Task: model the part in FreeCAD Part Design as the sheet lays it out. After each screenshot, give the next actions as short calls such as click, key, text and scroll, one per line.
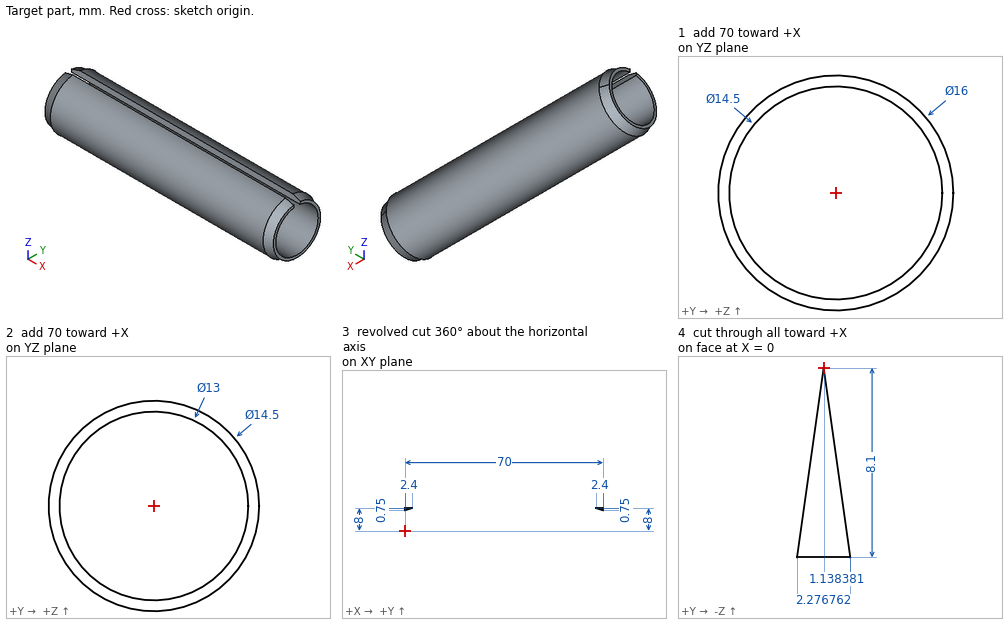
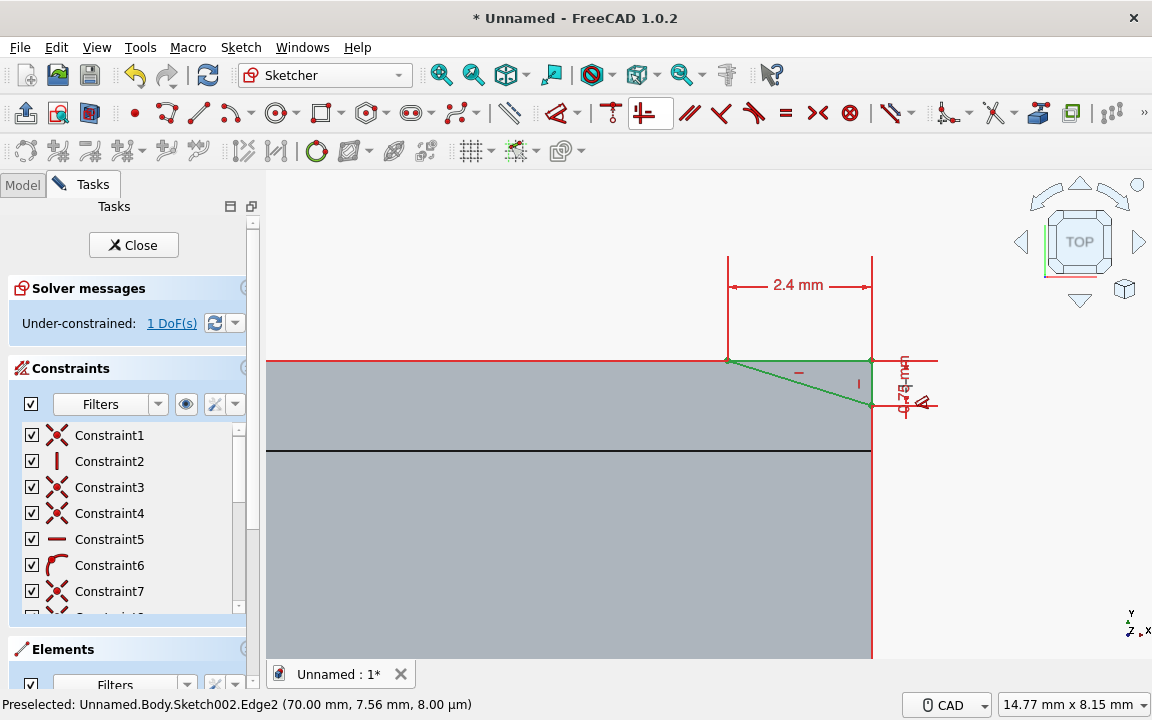
scroll(873, 391, down, 11)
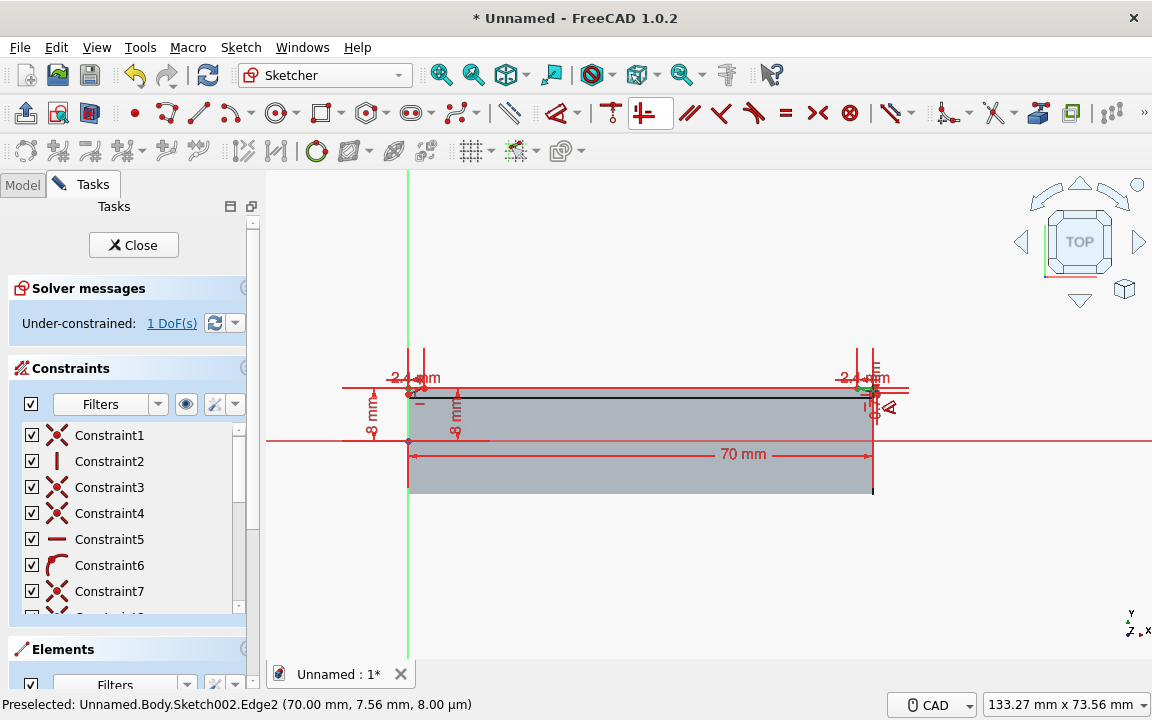
scroll(408, 390, up, 11)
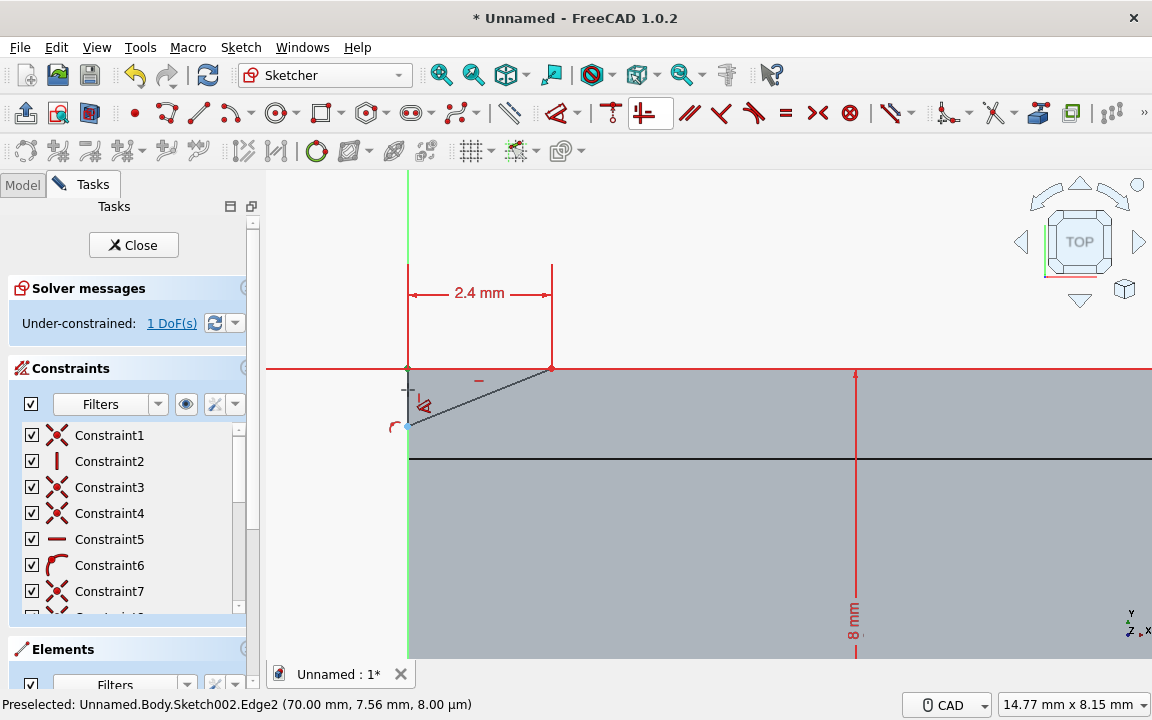
click(408, 386)
click(374, 398)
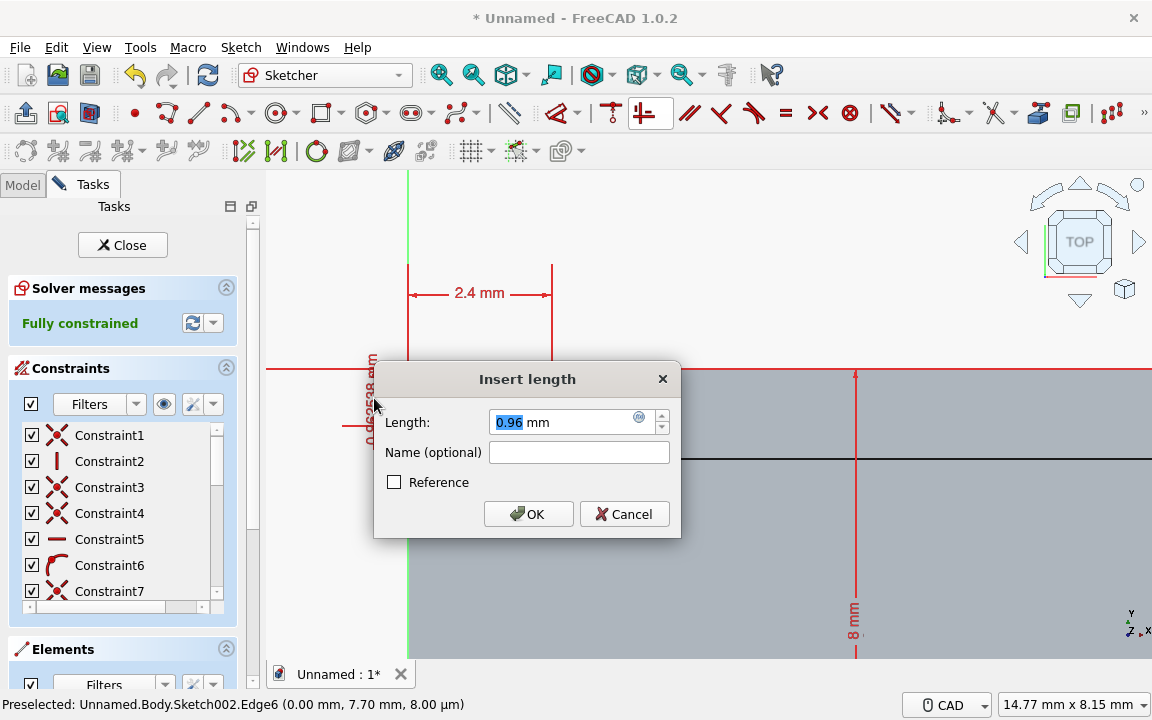
text(0.75)
key(Return)
key(Escape)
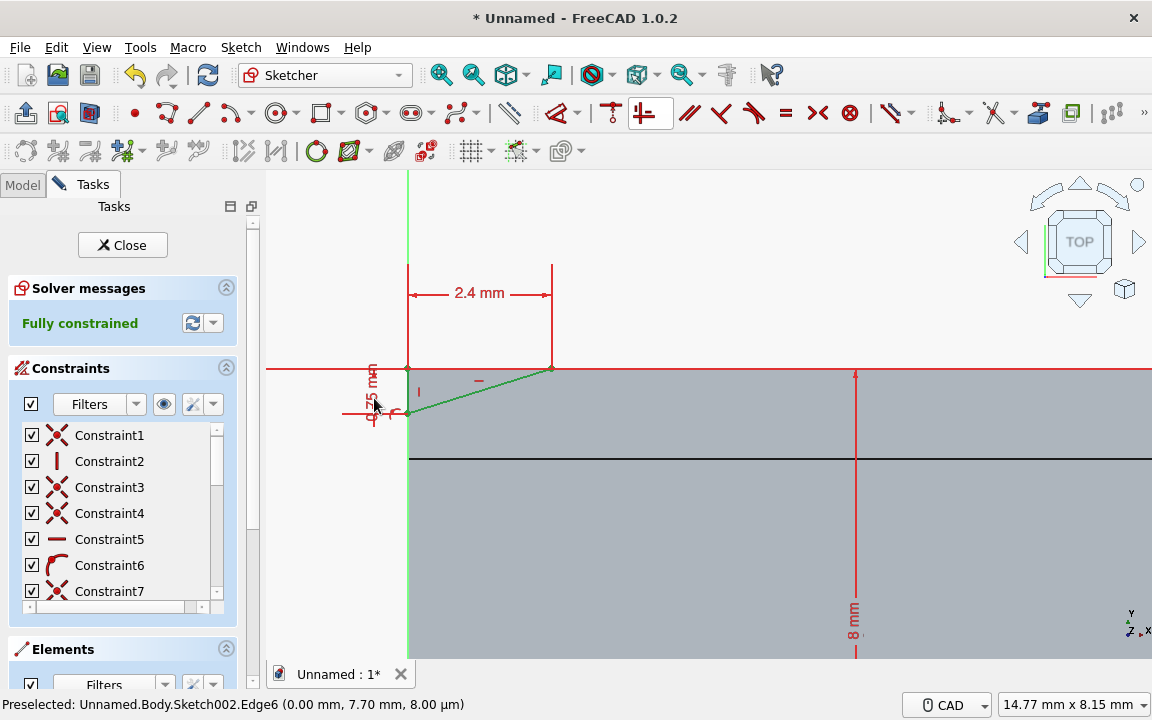
click(123, 245)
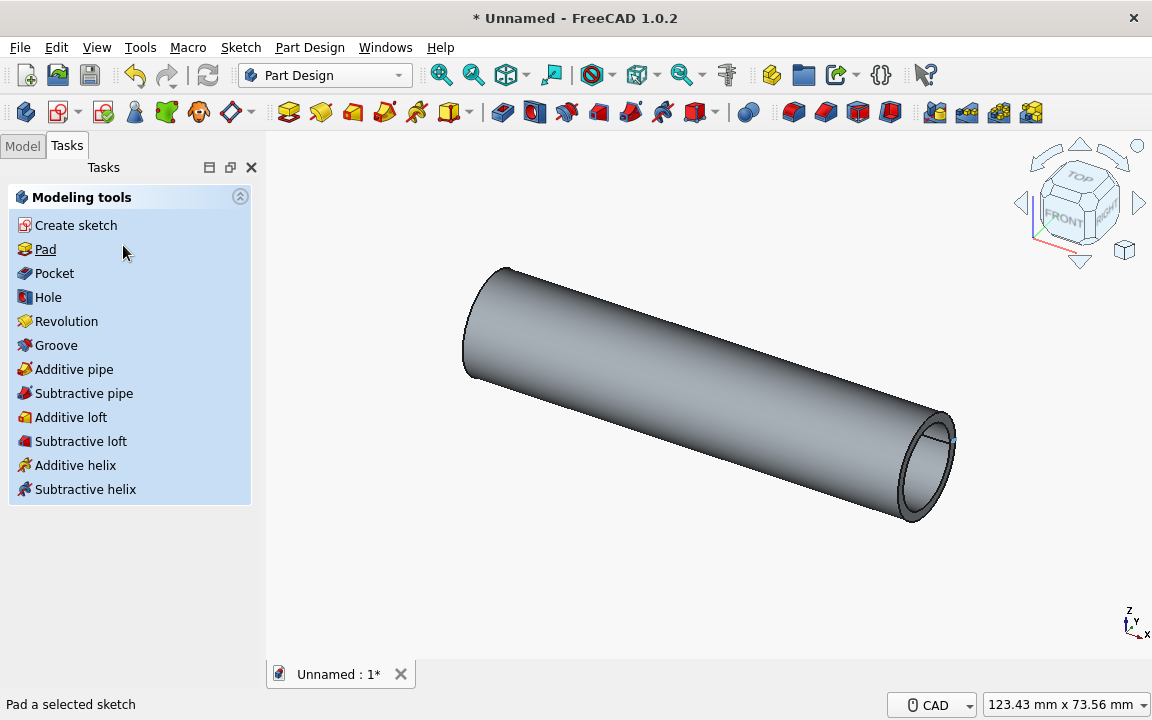
click(568, 112)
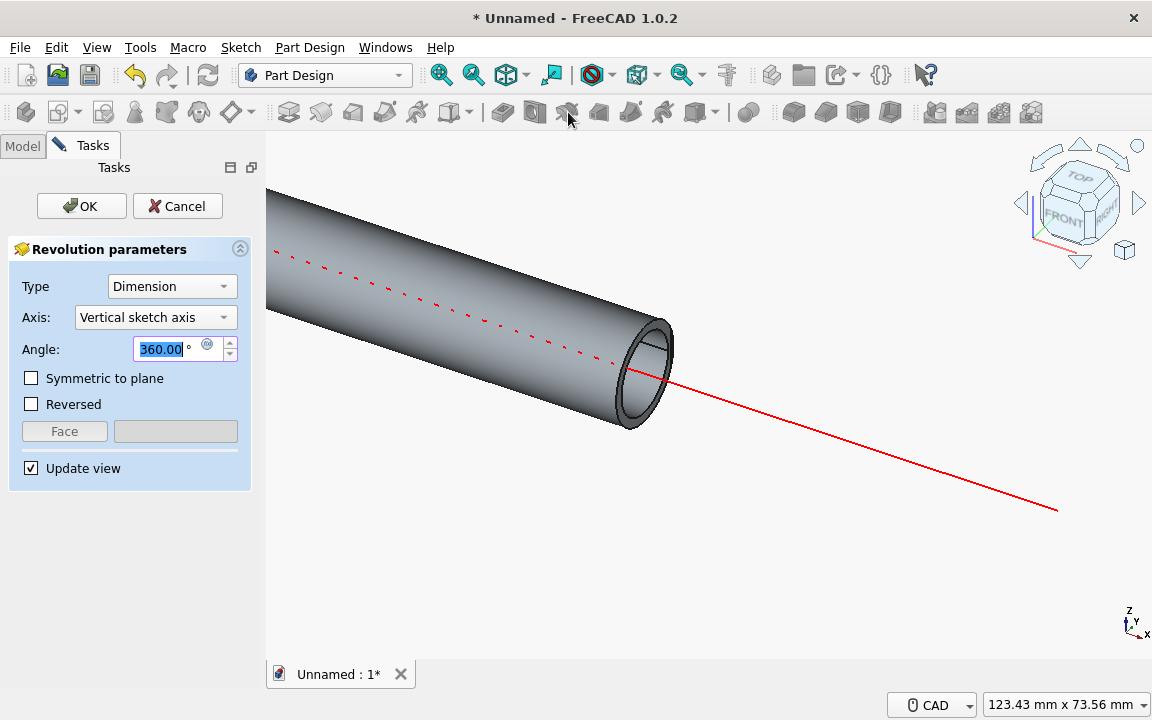
click(156, 318)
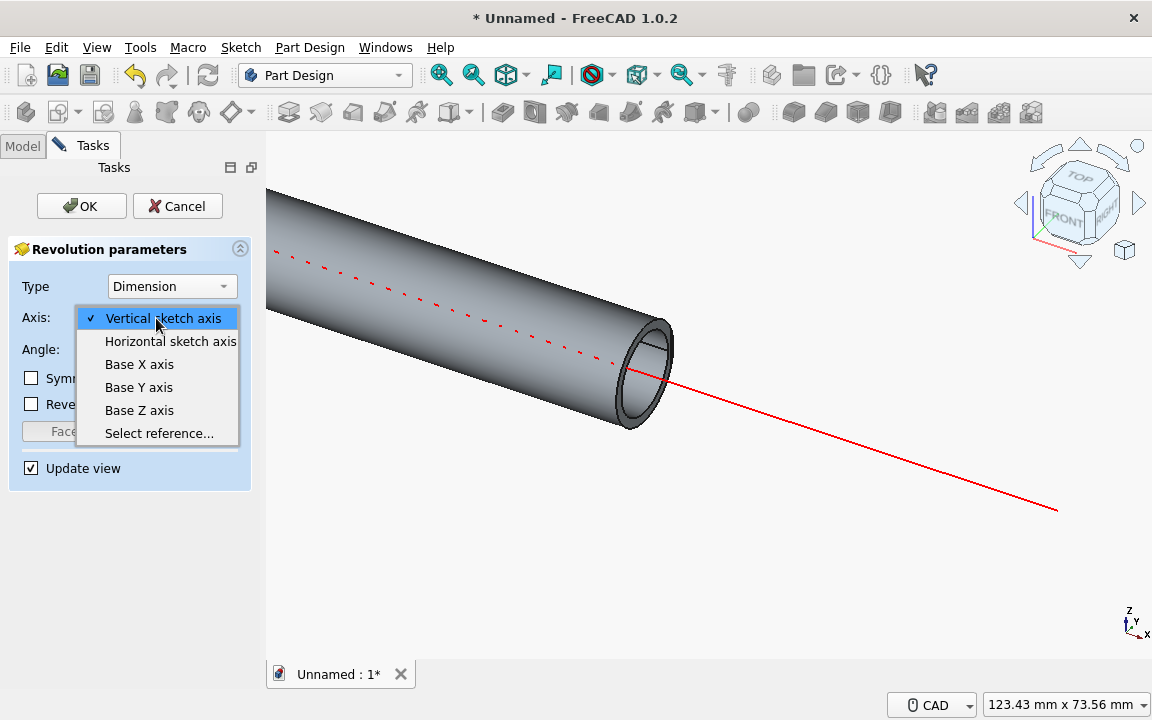
click(156, 342)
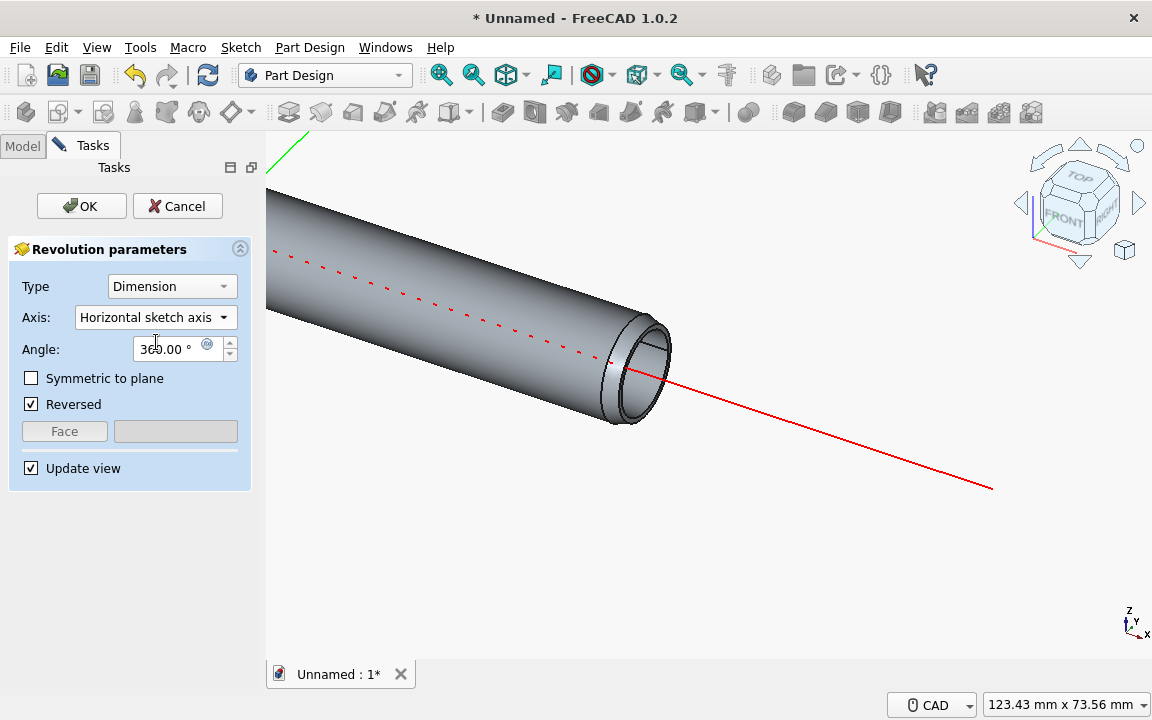
click(82, 206)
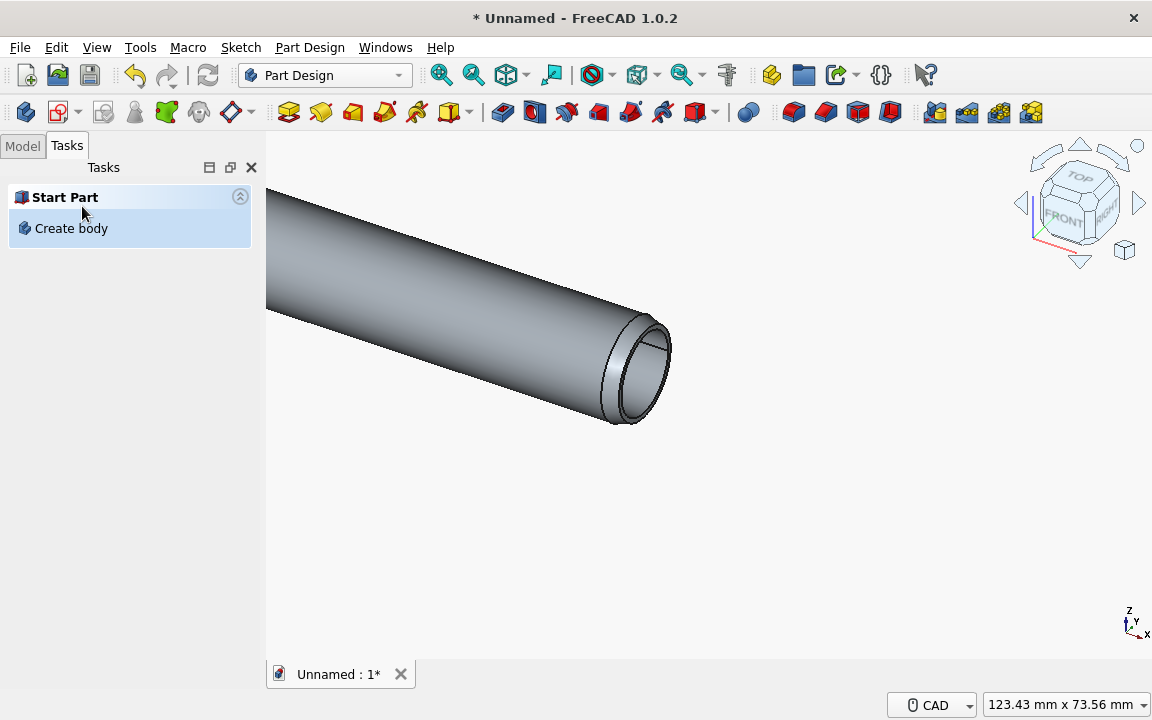
click(442, 76)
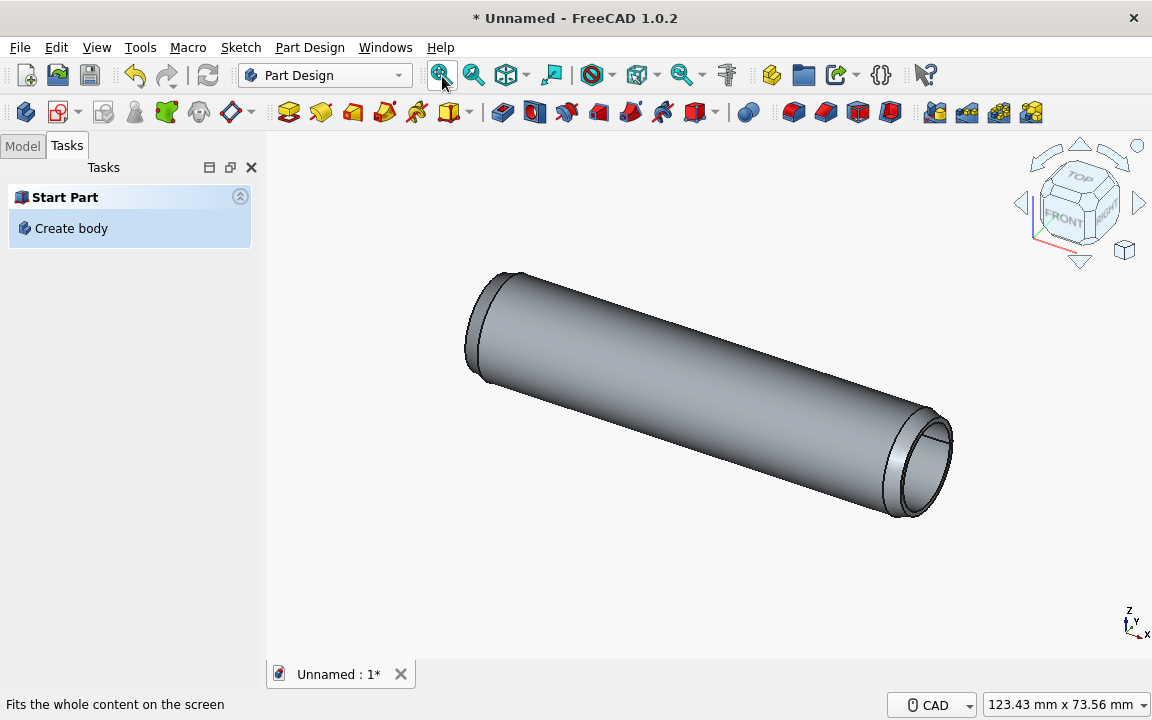
key(6)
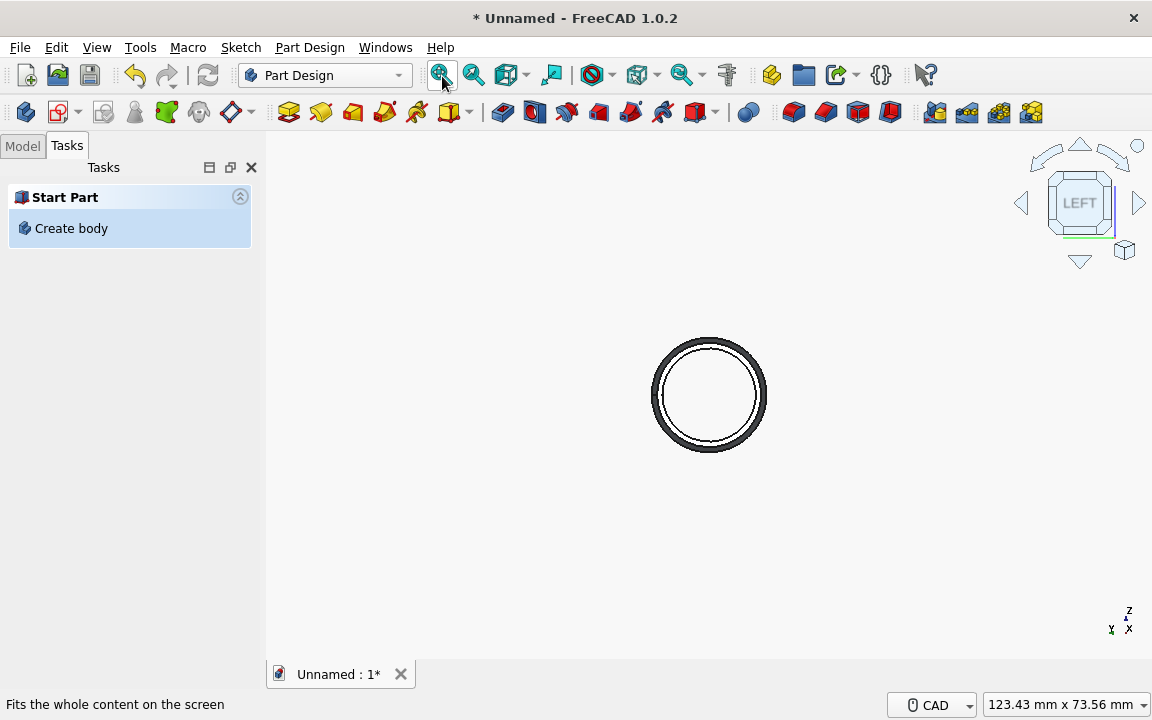
click(442, 76)